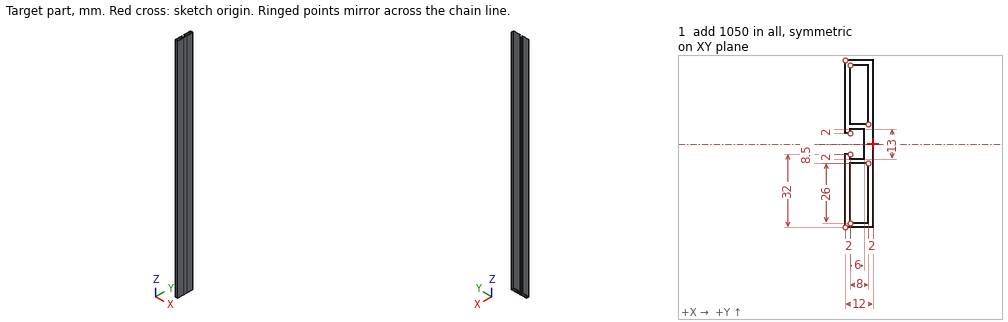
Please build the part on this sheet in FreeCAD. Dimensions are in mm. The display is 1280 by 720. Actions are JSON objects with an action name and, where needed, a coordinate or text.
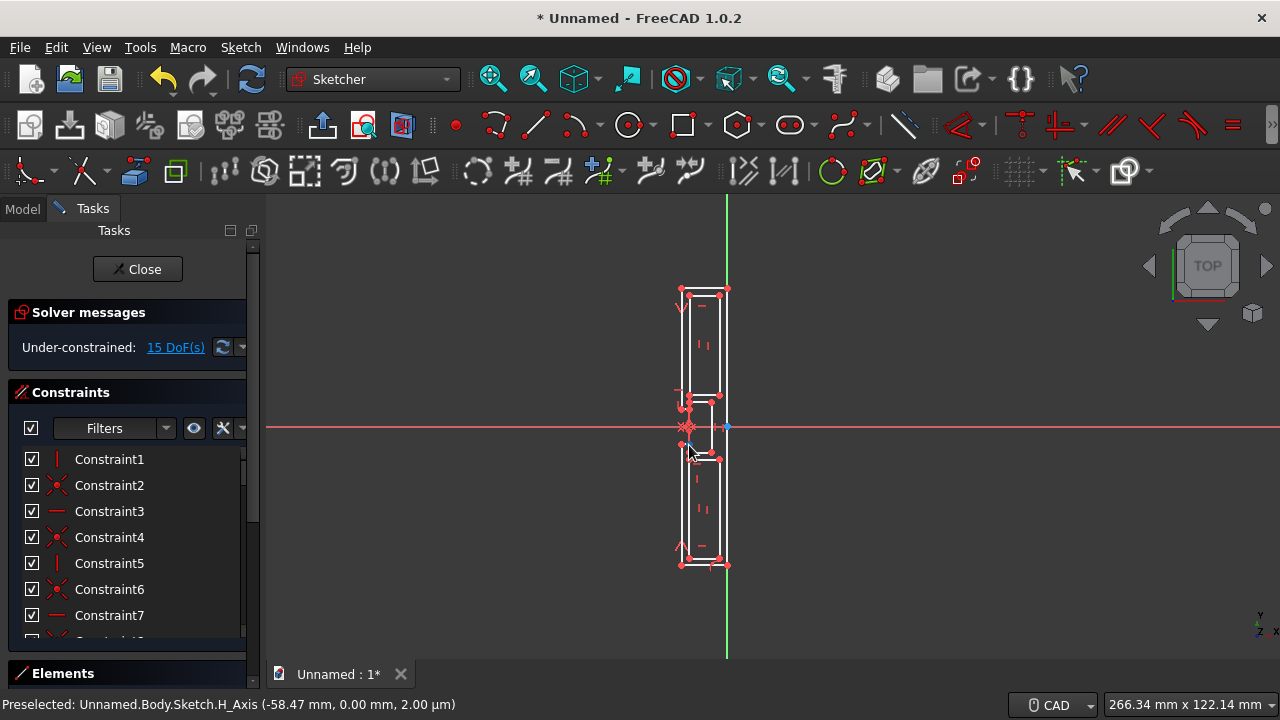
{"action": "left_click", "coordinate": [689, 559]}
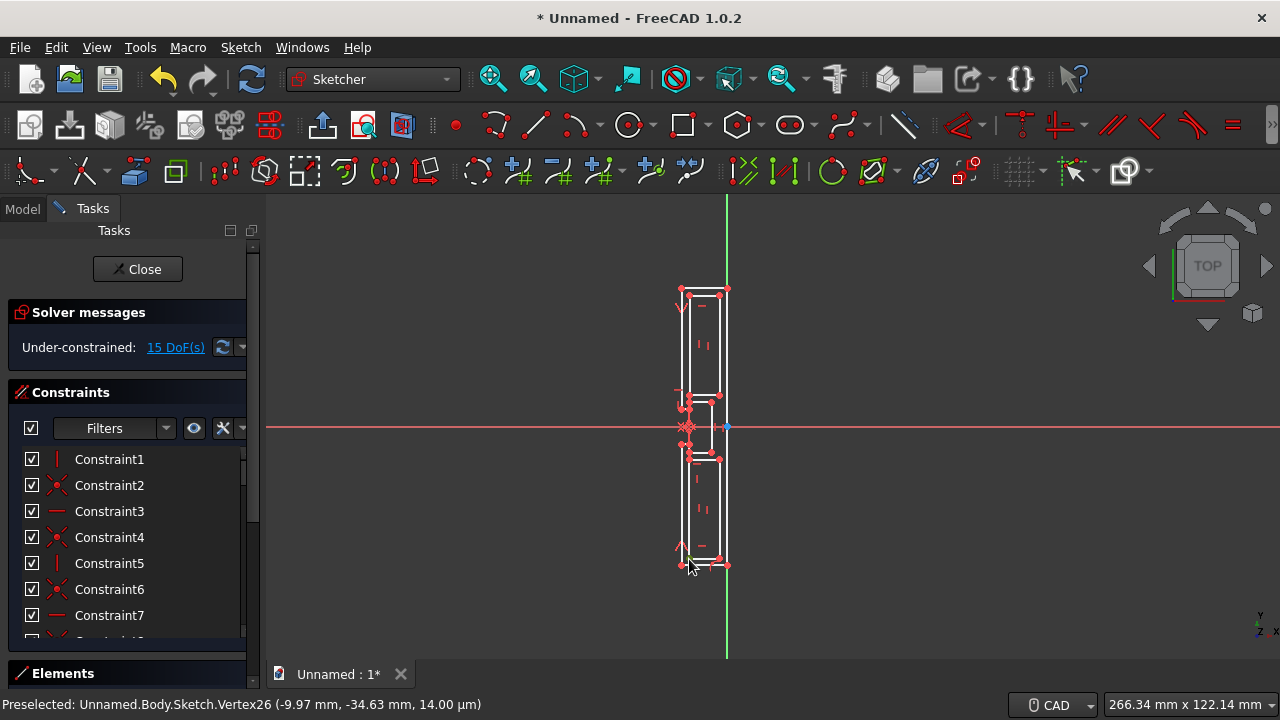
{"action": "left_click", "coordinate": [690, 296]}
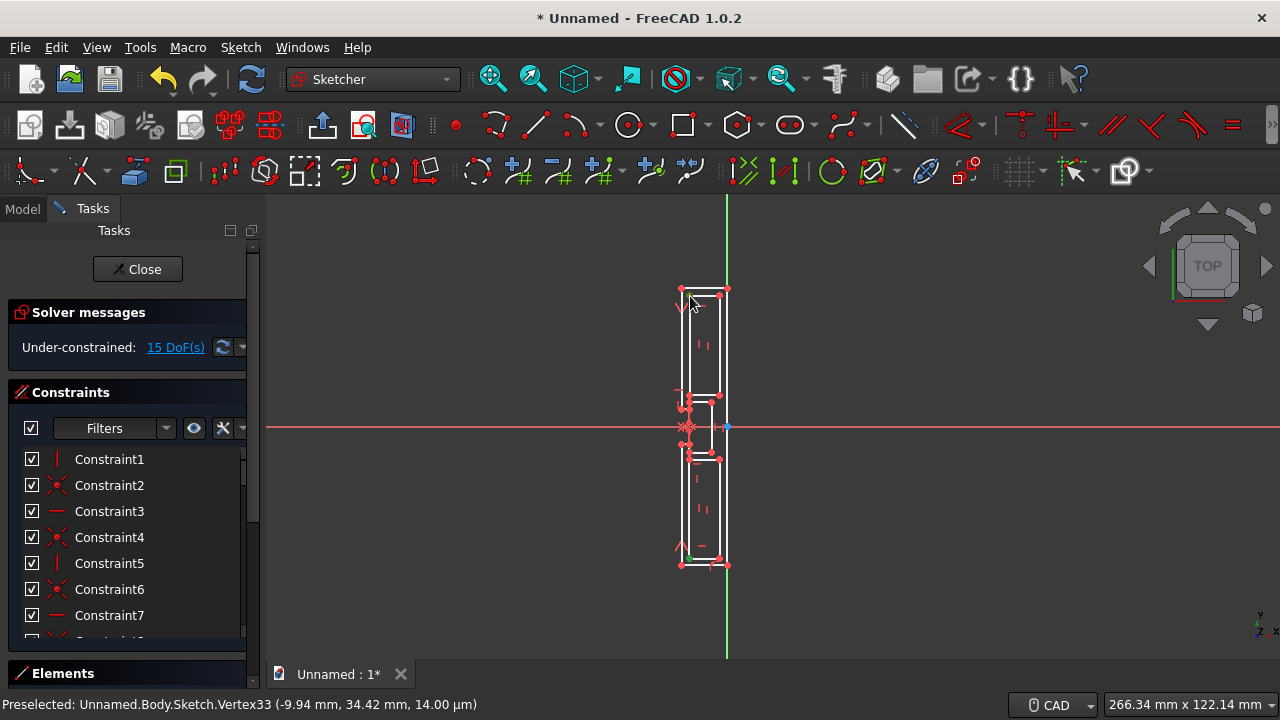
{"action": "left_click", "coordinate": [353, 427]}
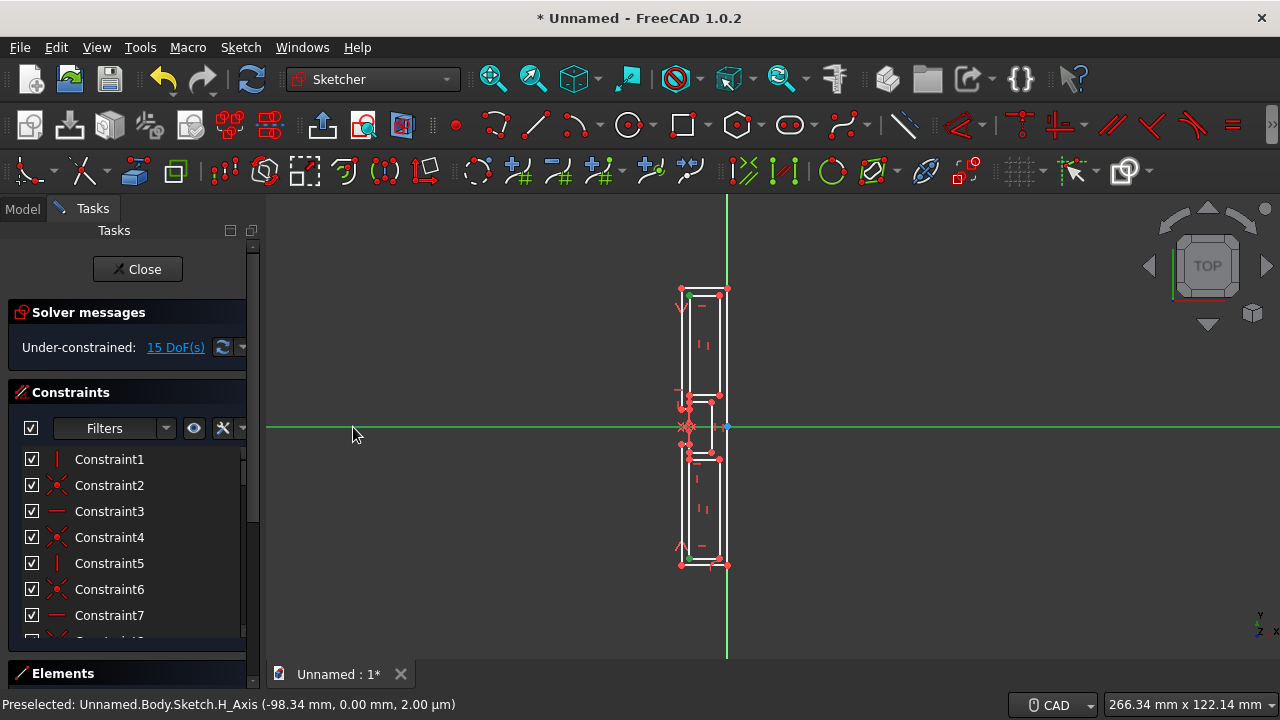
{"action": "key", "text": "s"}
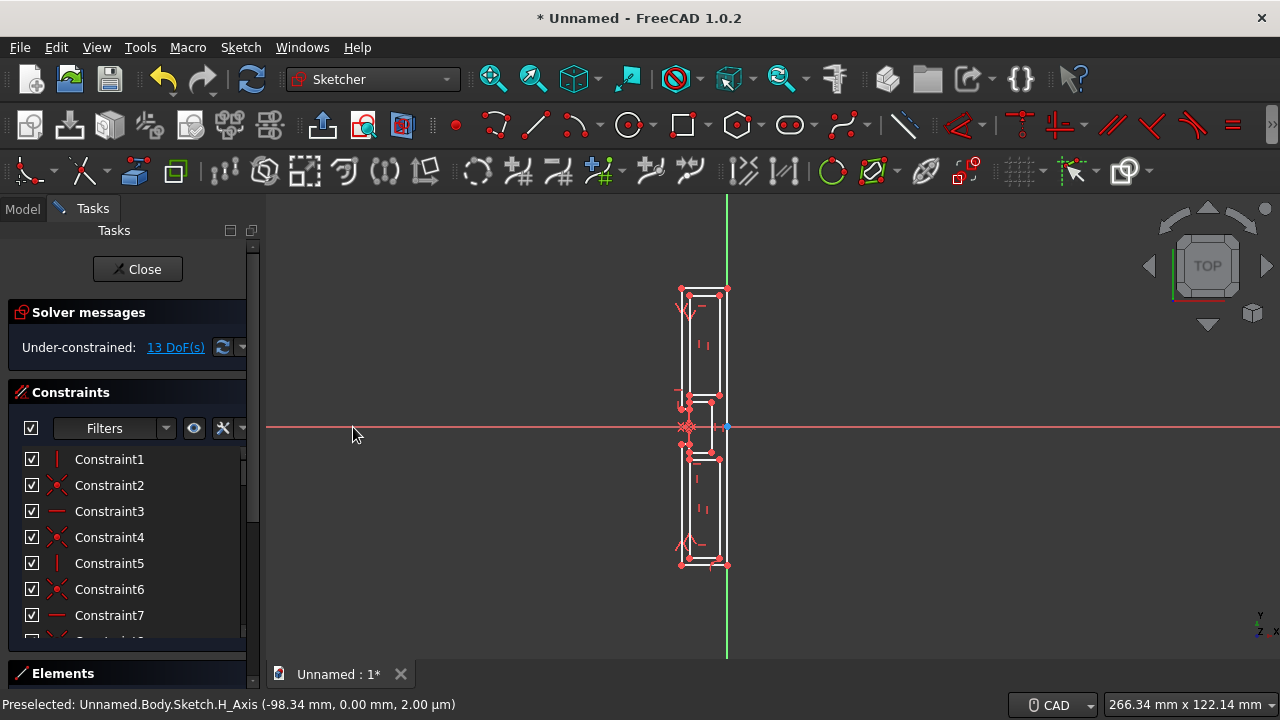
{"action": "left_click", "coordinate": [720, 460]}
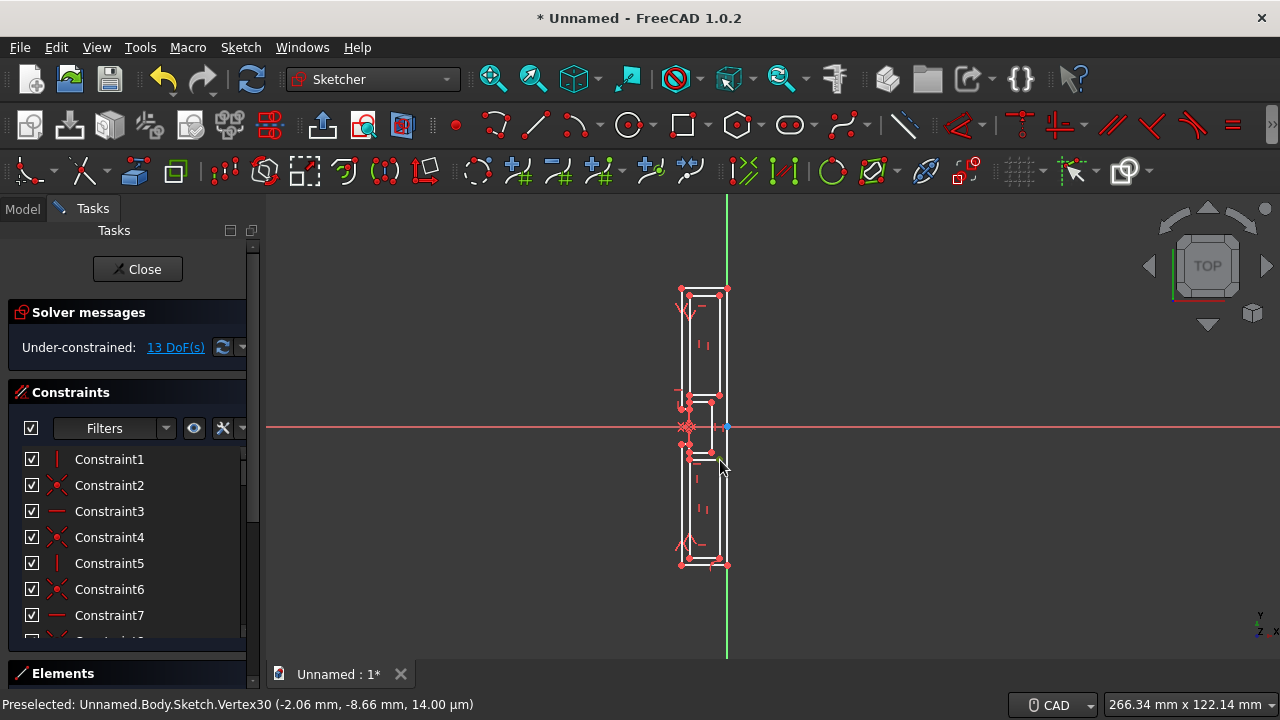
{"action": "left_click", "coordinate": [720, 395]}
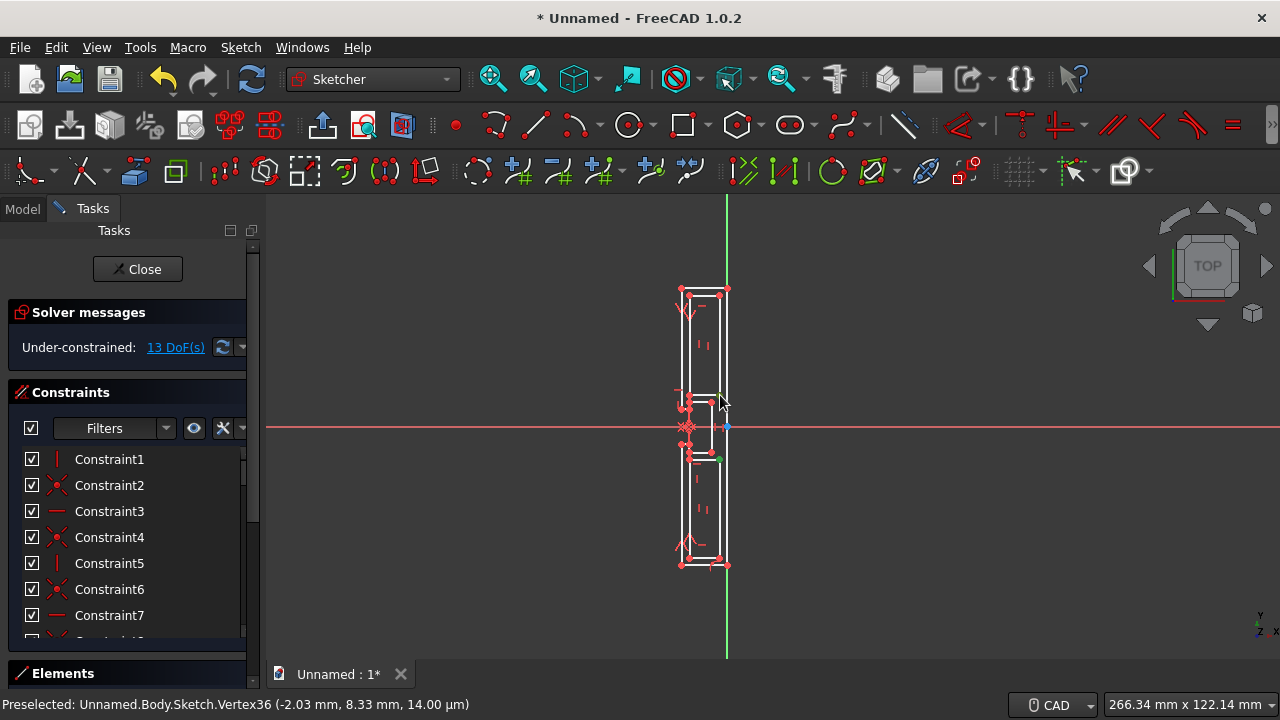
{"action": "left_click", "coordinate": [353, 427]}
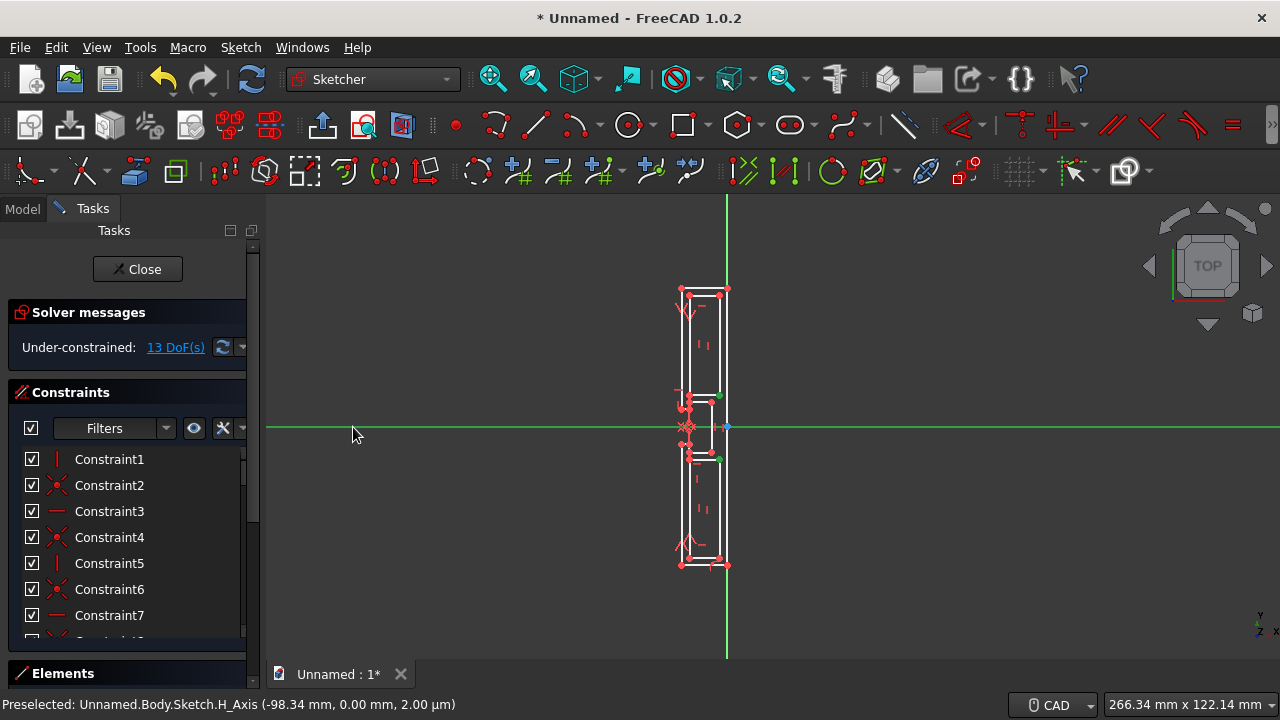
{"action": "key", "text": "s"}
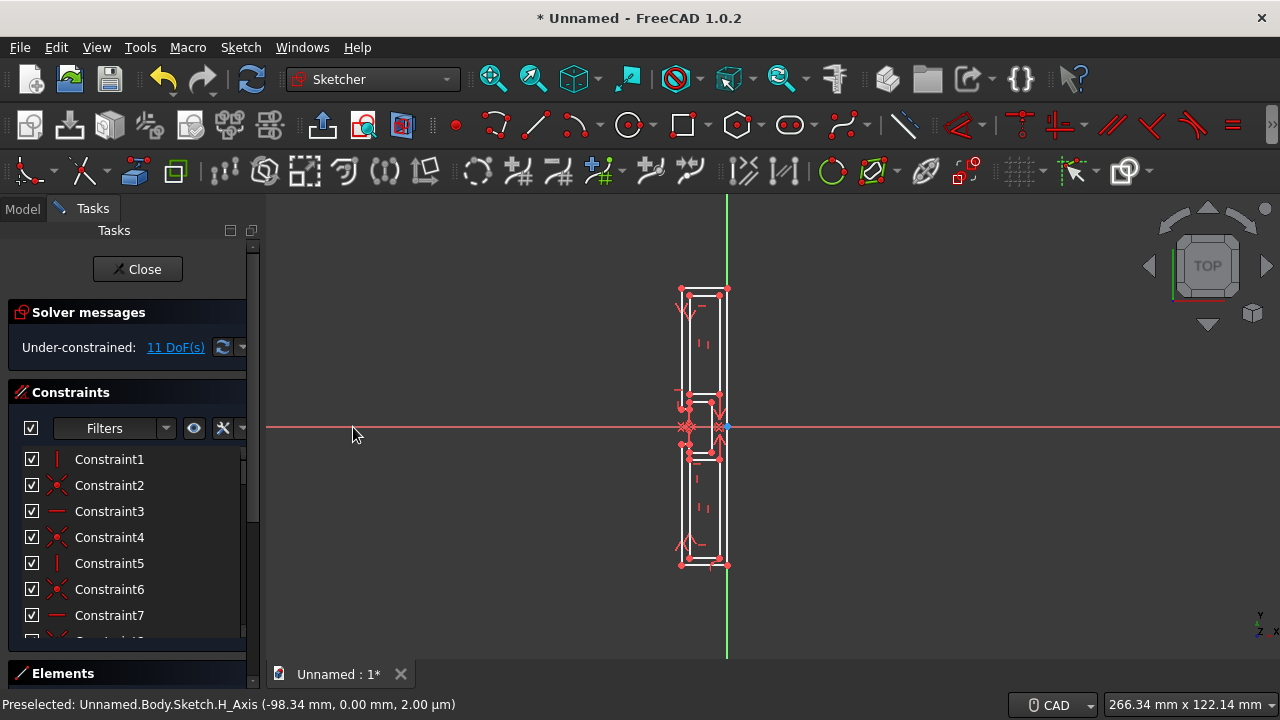
{"action": "left_click", "coordinate": [958, 126]}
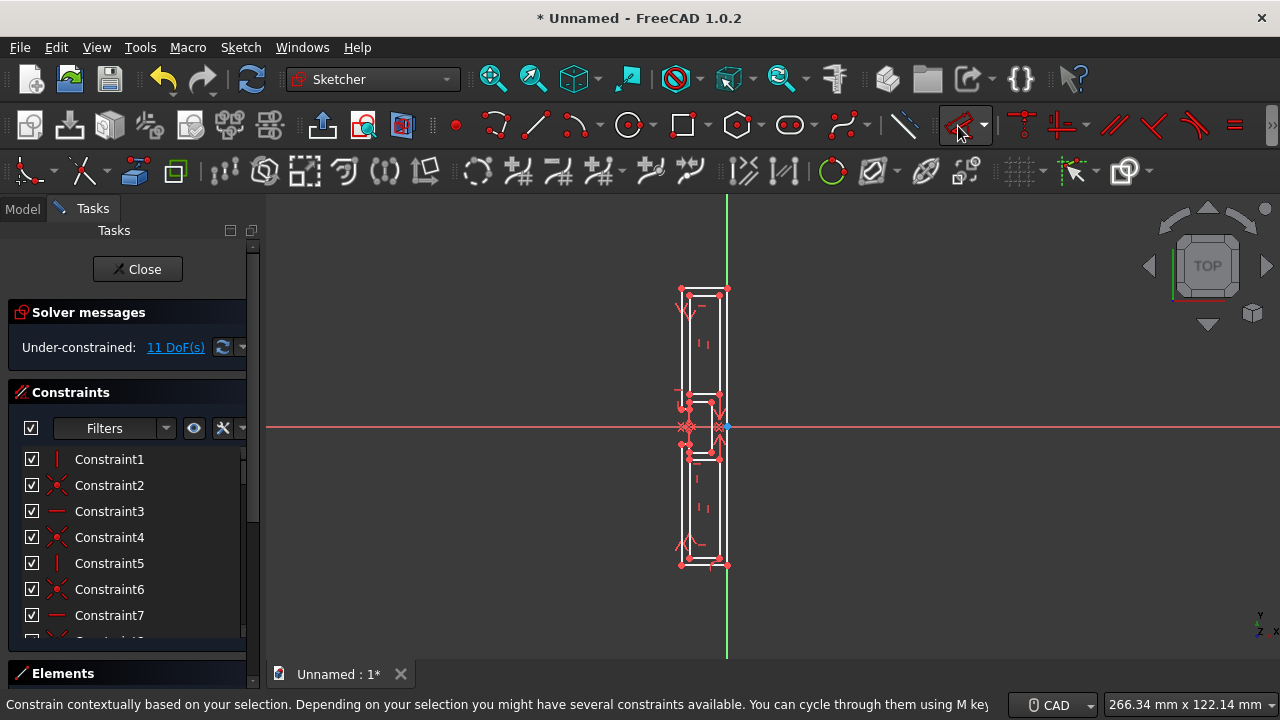
{"action": "scroll", "coordinate": [703, 453], "scroll_direction": "up", "scroll_amount": 4}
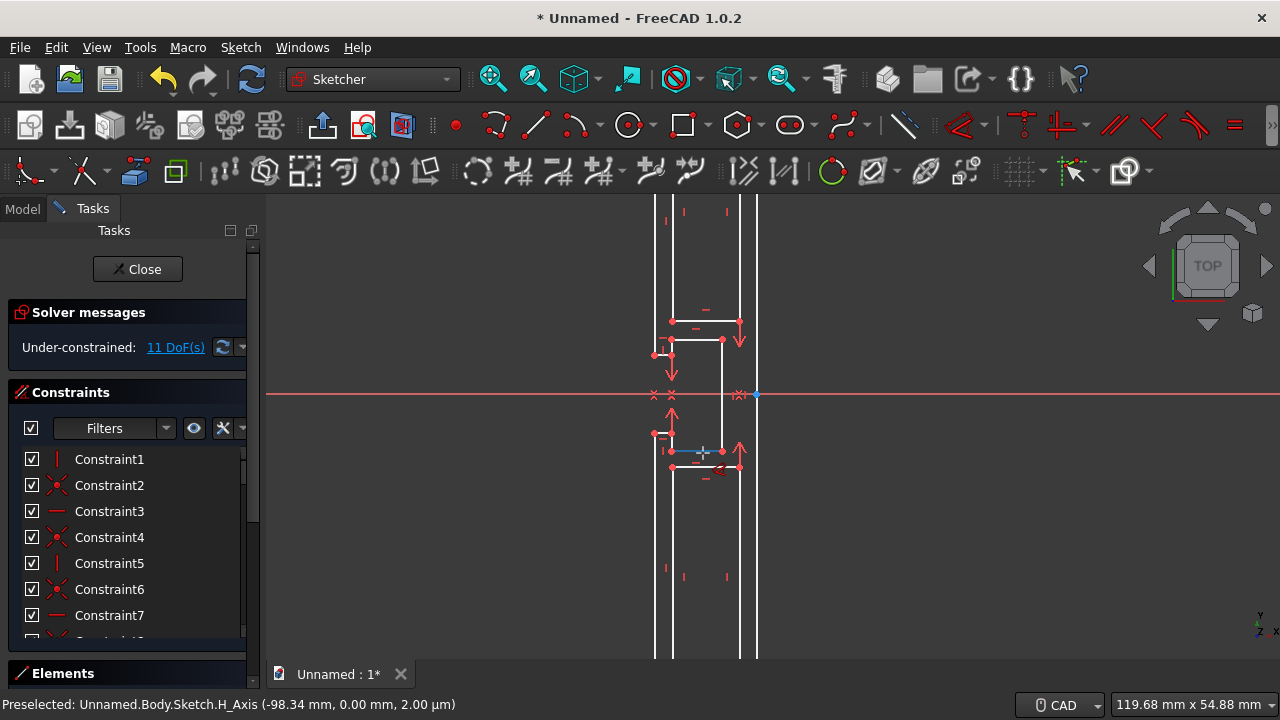
{"action": "left_click", "coordinate": [702, 451]}
{"action": "left_click", "coordinate": [697, 485]}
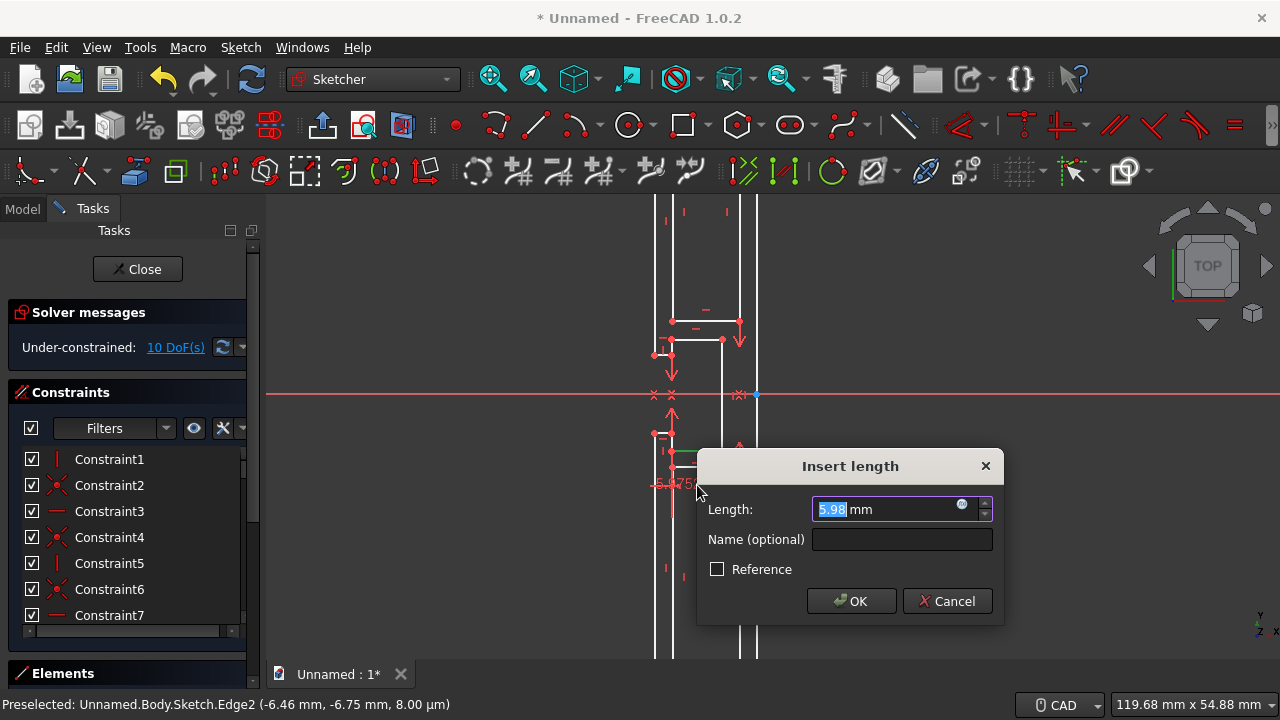
{"action": "type", "text": "6"}
{"action": "key", "text": "Return"}